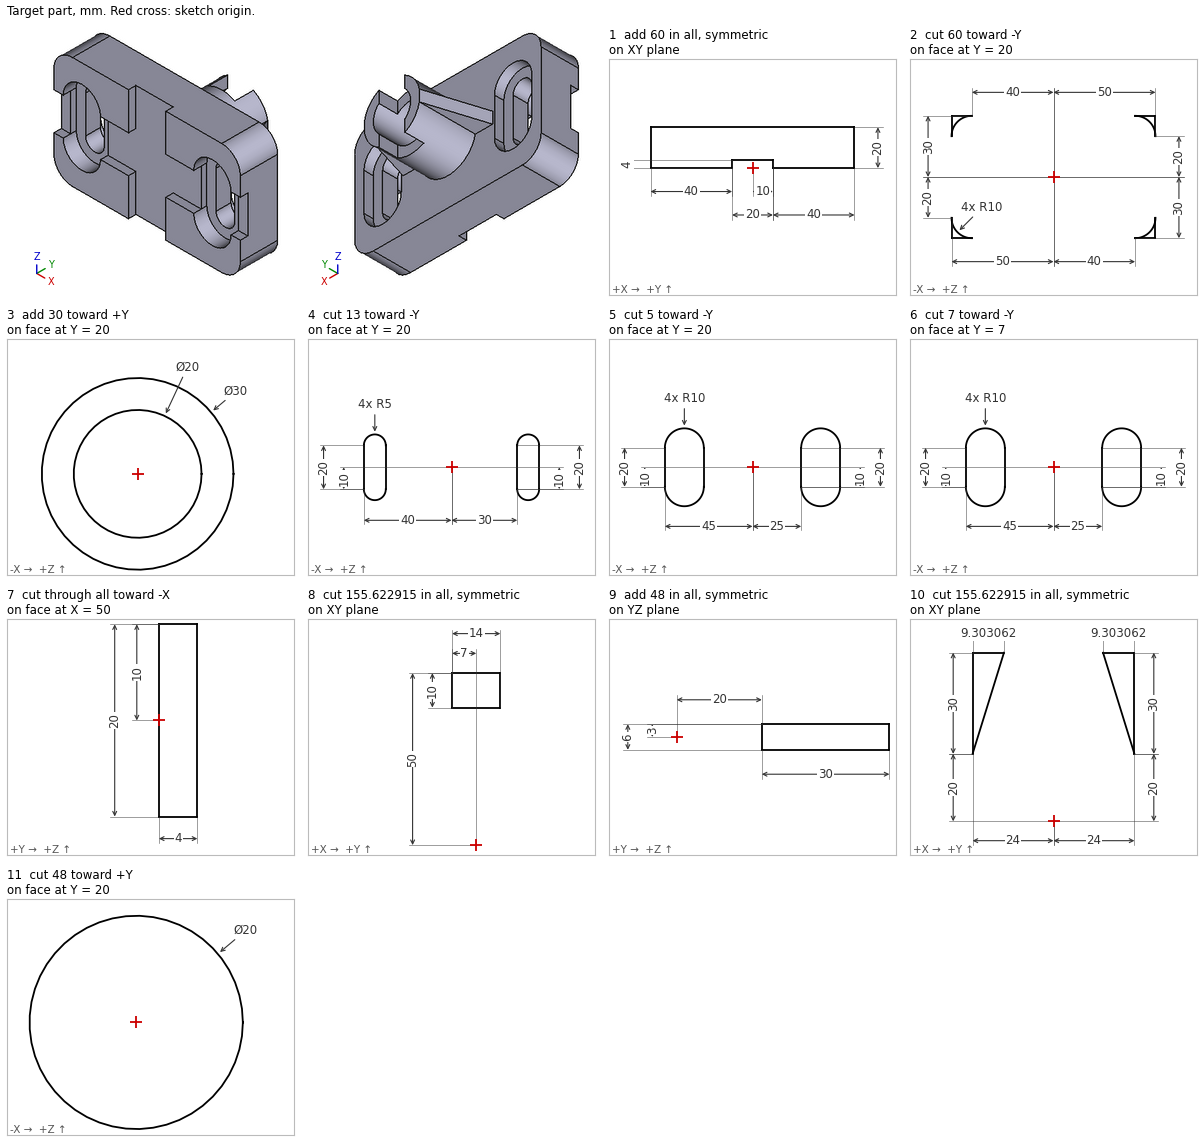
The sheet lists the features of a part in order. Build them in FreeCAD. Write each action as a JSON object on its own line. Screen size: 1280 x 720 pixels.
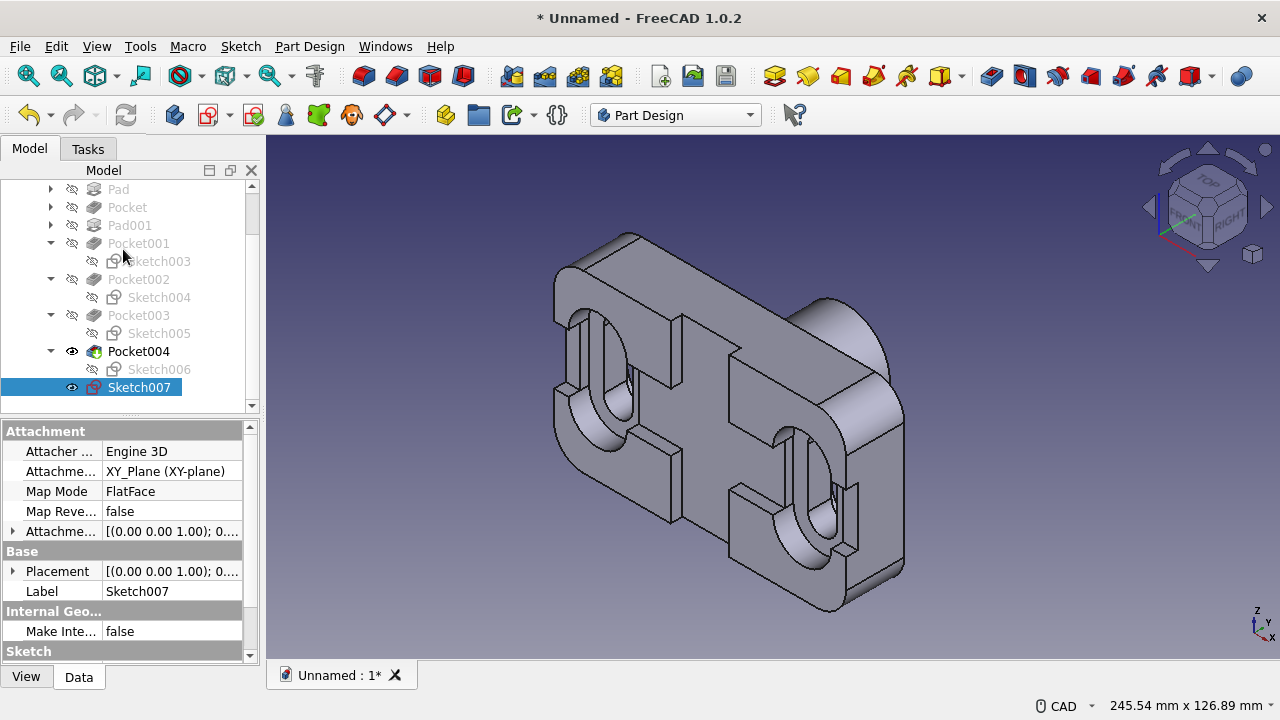
{"action": "left_click", "coordinate": [992, 76]}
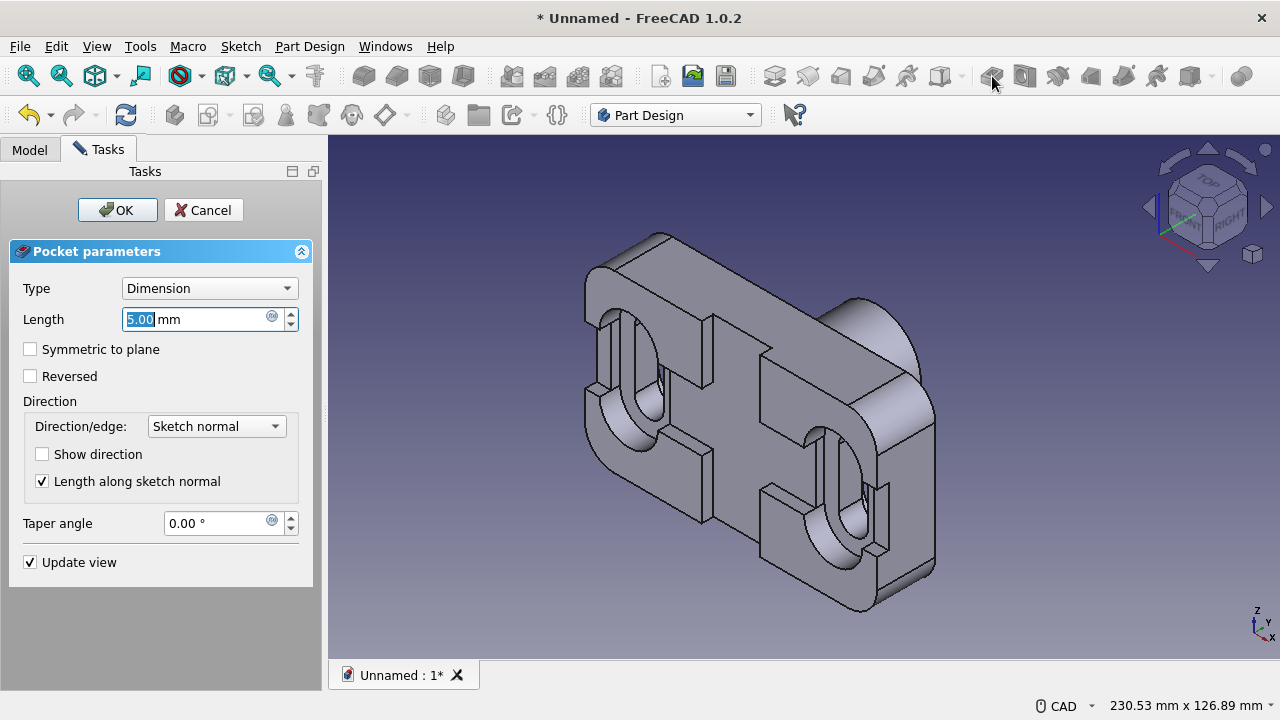
{"action": "type", "text": "155.622915"}
{"action": "key", "text": "Tab"}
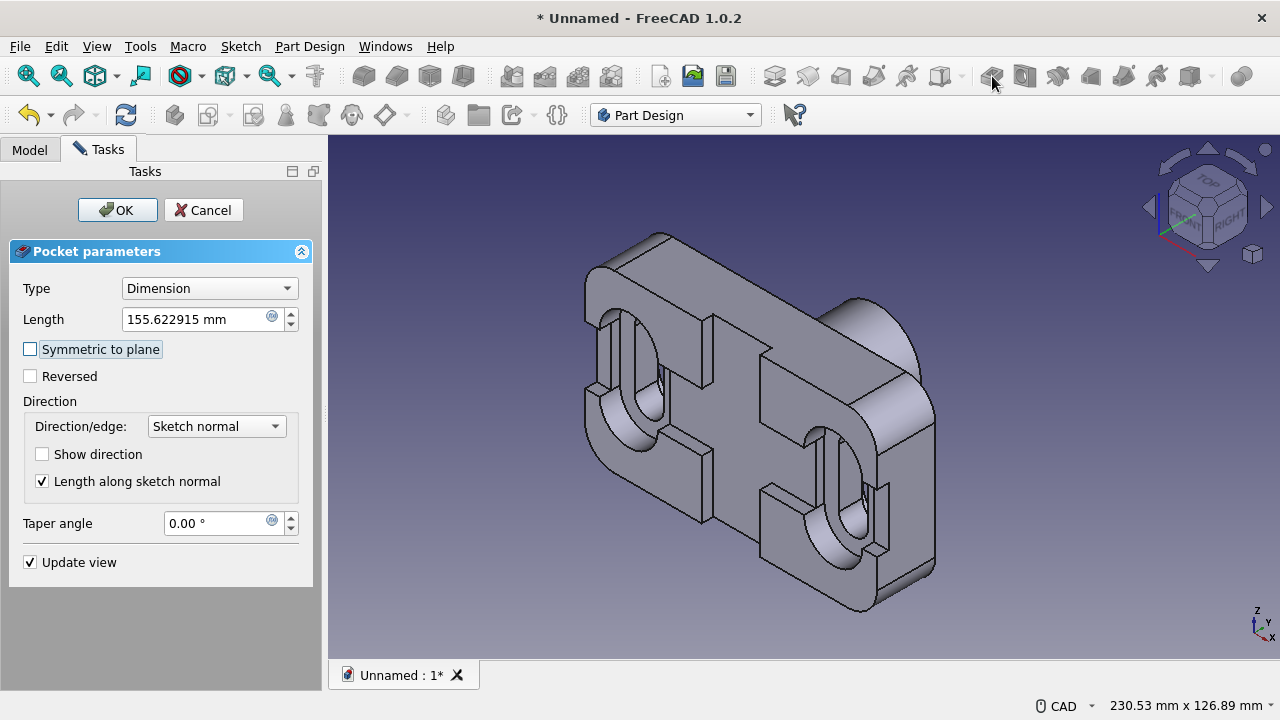
{"action": "left_click", "coordinate": [31, 349]}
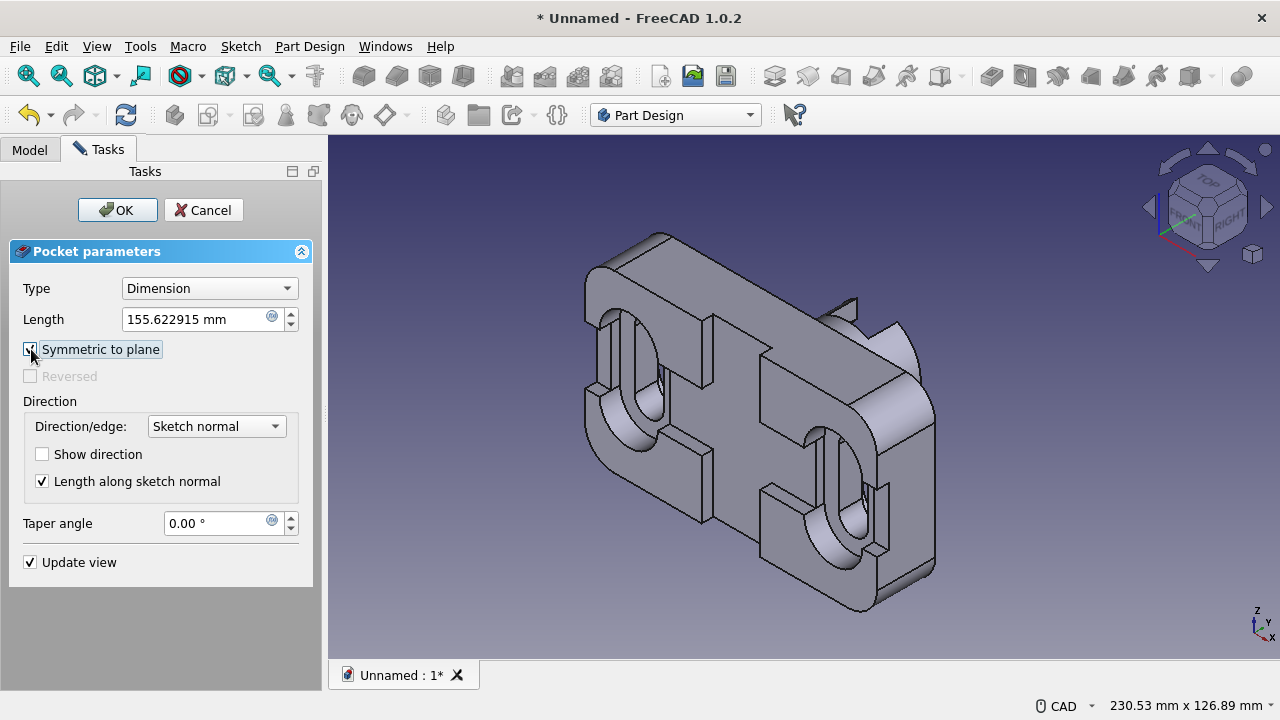
{"action": "left_click", "coordinate": [118, 210]}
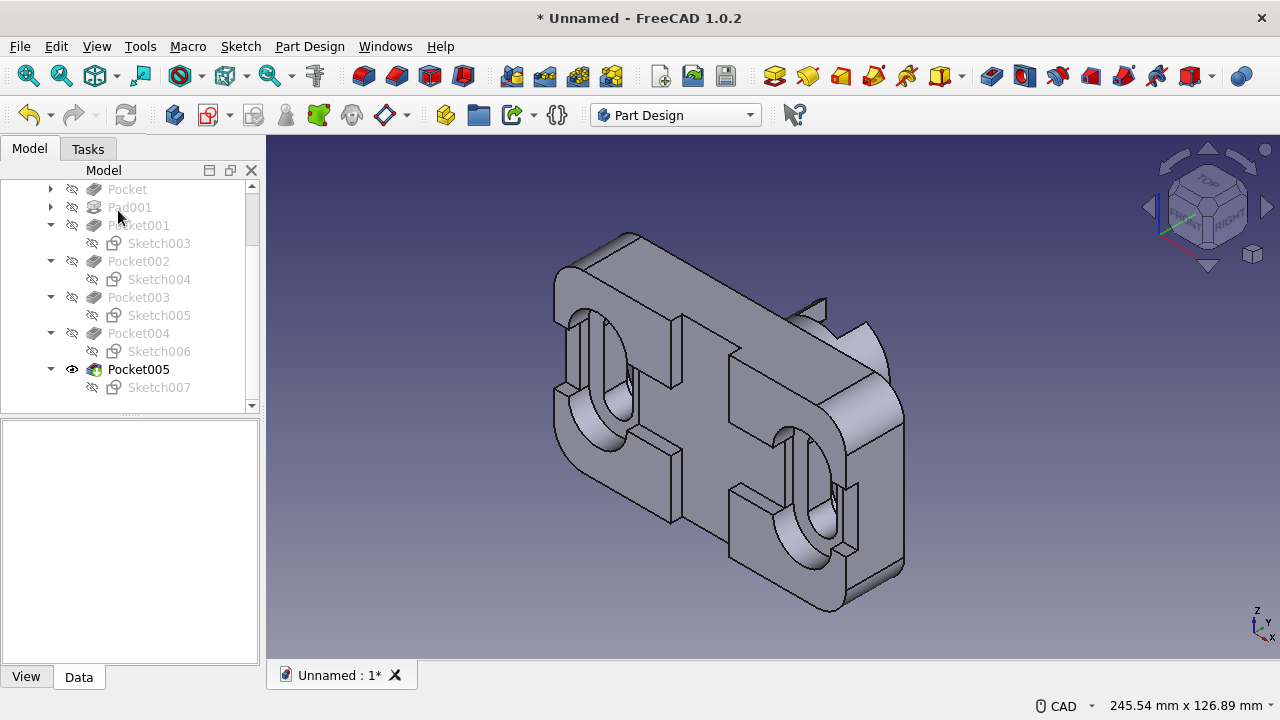
{"action": "left_click", "coordinate": [208, 116]}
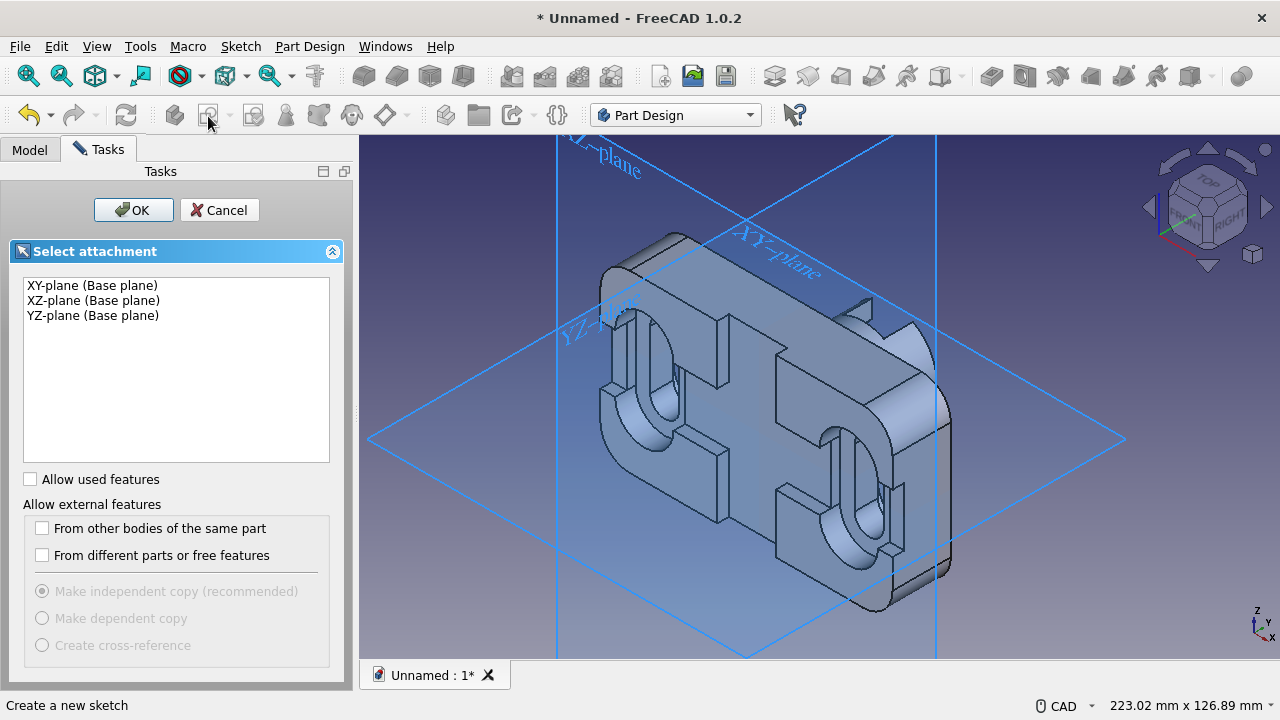
{"action": "left_click", "coordinate": [84, 316]}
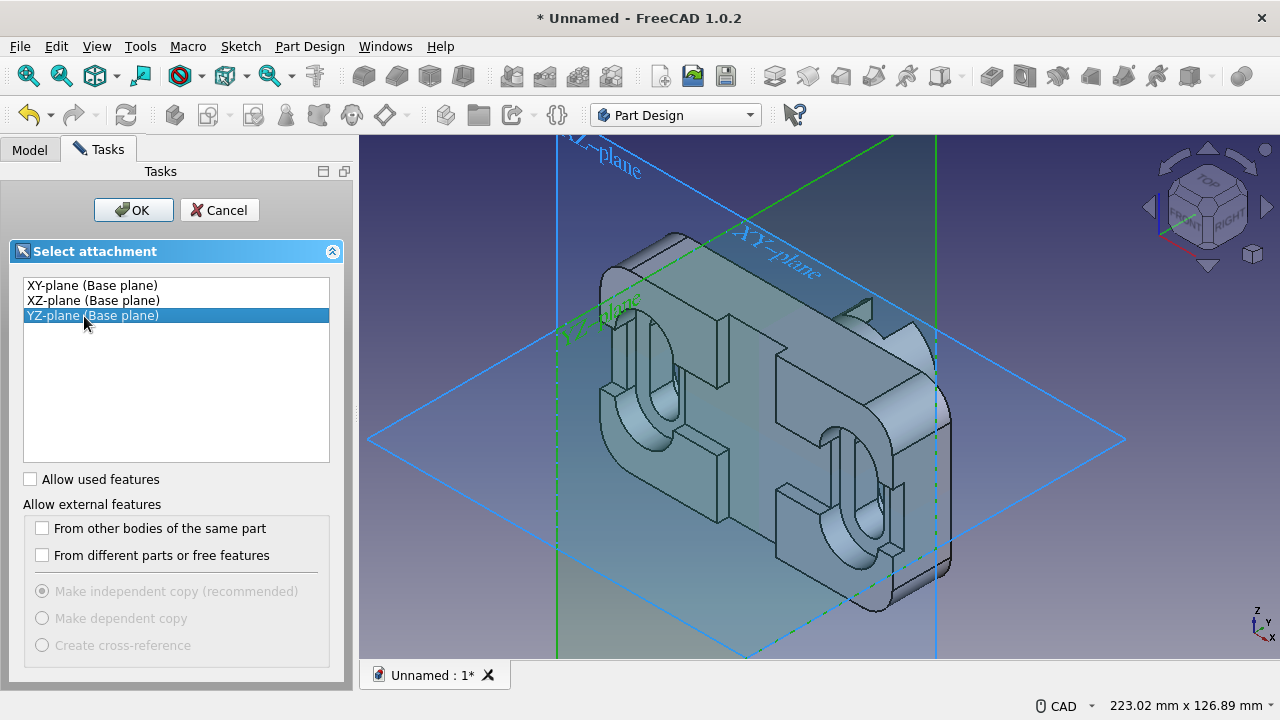
{"action": "left_click", "coordinate": [134, 210]}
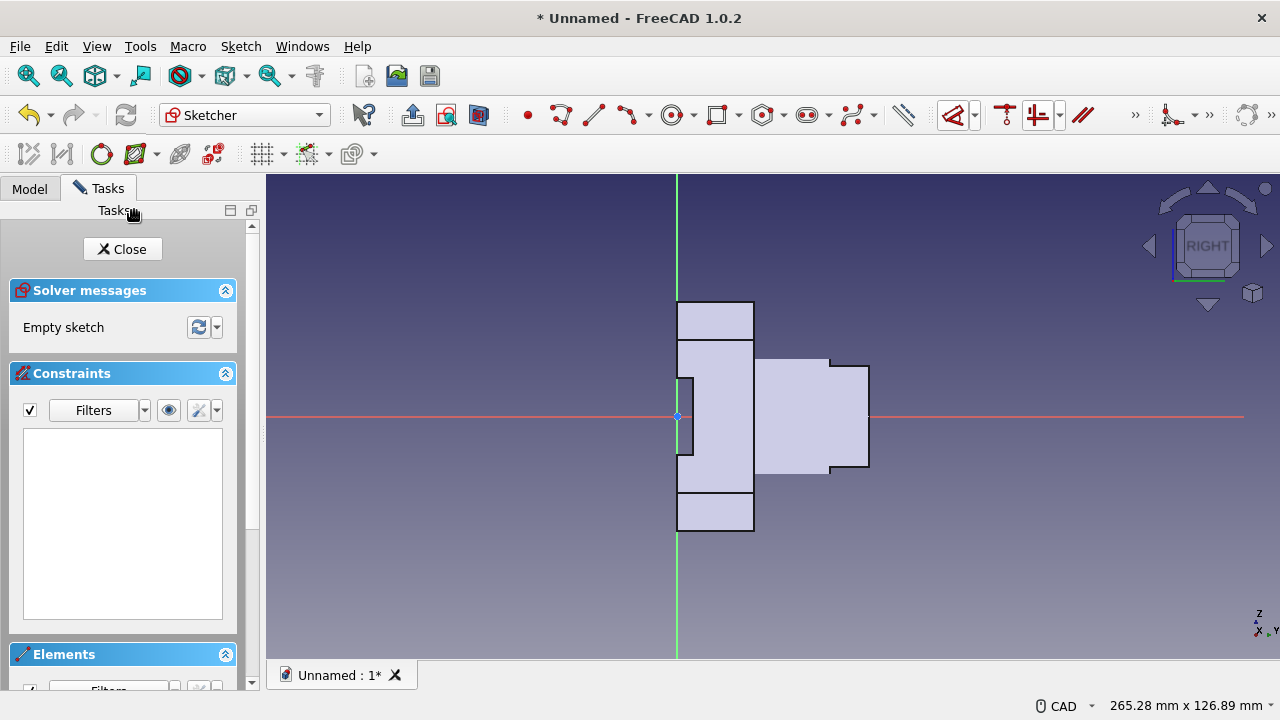
{"action": "key", "text": "q s"}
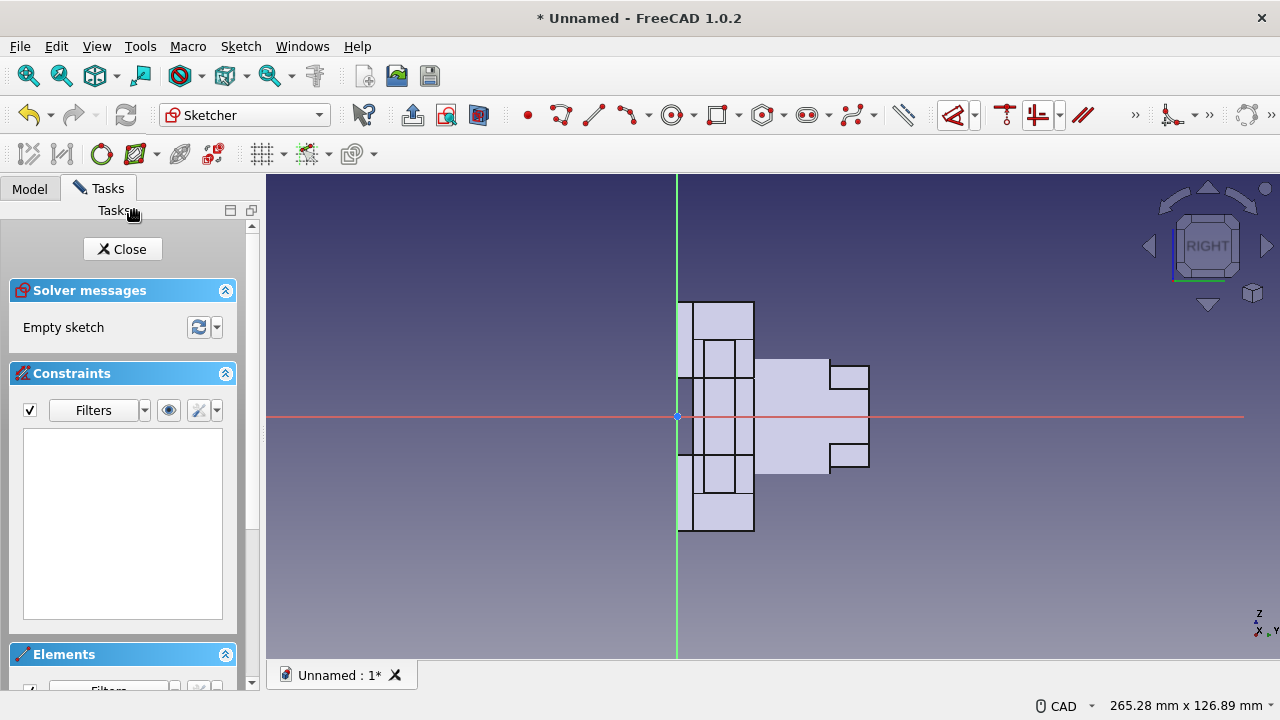
{"action": "scroll", "coordinate": [803, 416], "scroll_direction": "up", "scroll_amount": 6}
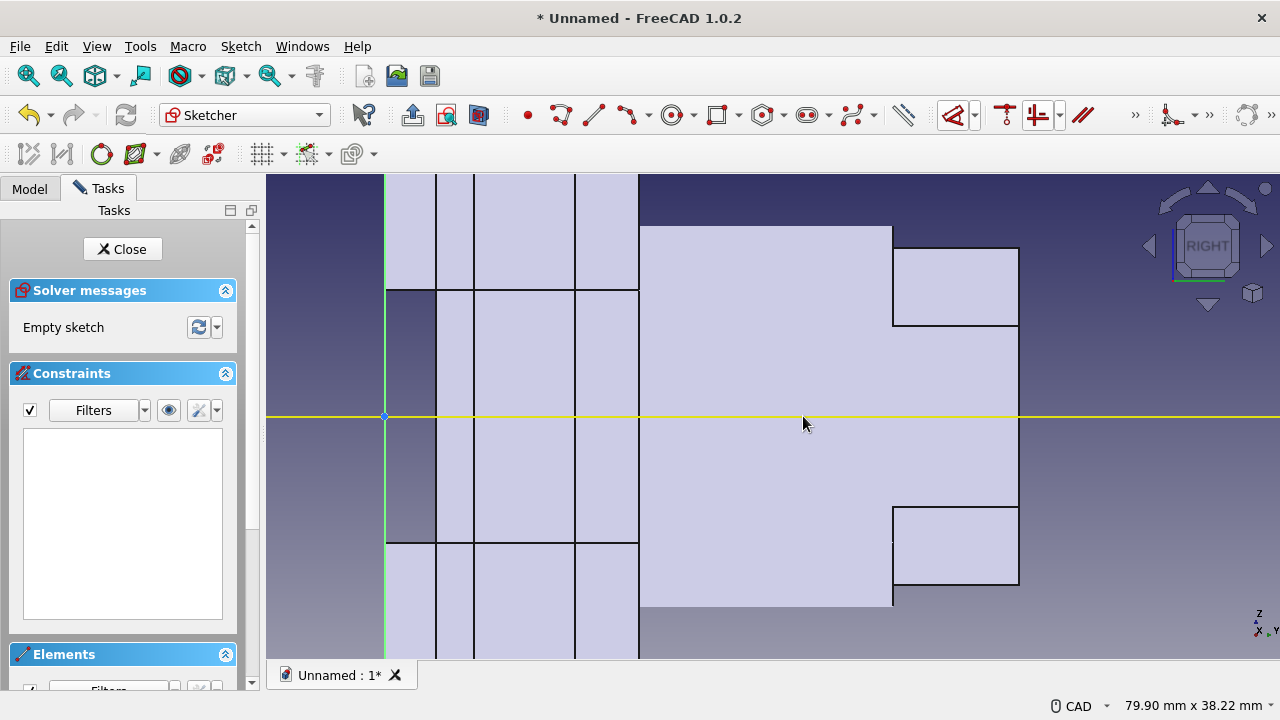
{"action": "key", "text": "g r"}